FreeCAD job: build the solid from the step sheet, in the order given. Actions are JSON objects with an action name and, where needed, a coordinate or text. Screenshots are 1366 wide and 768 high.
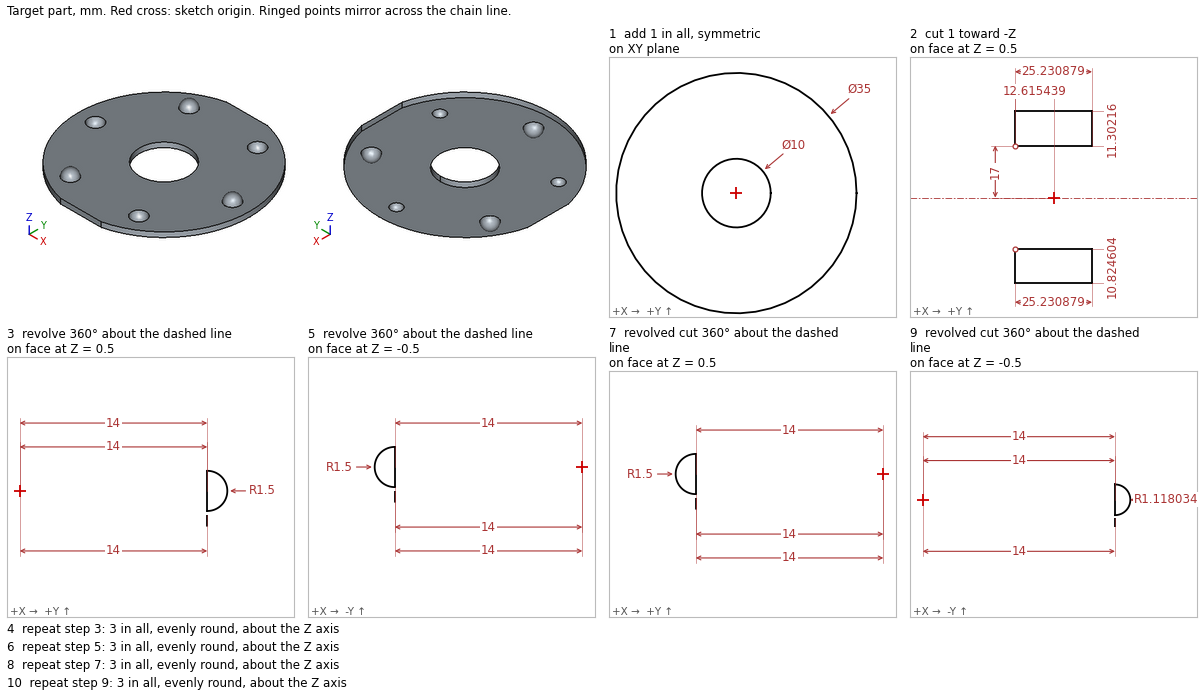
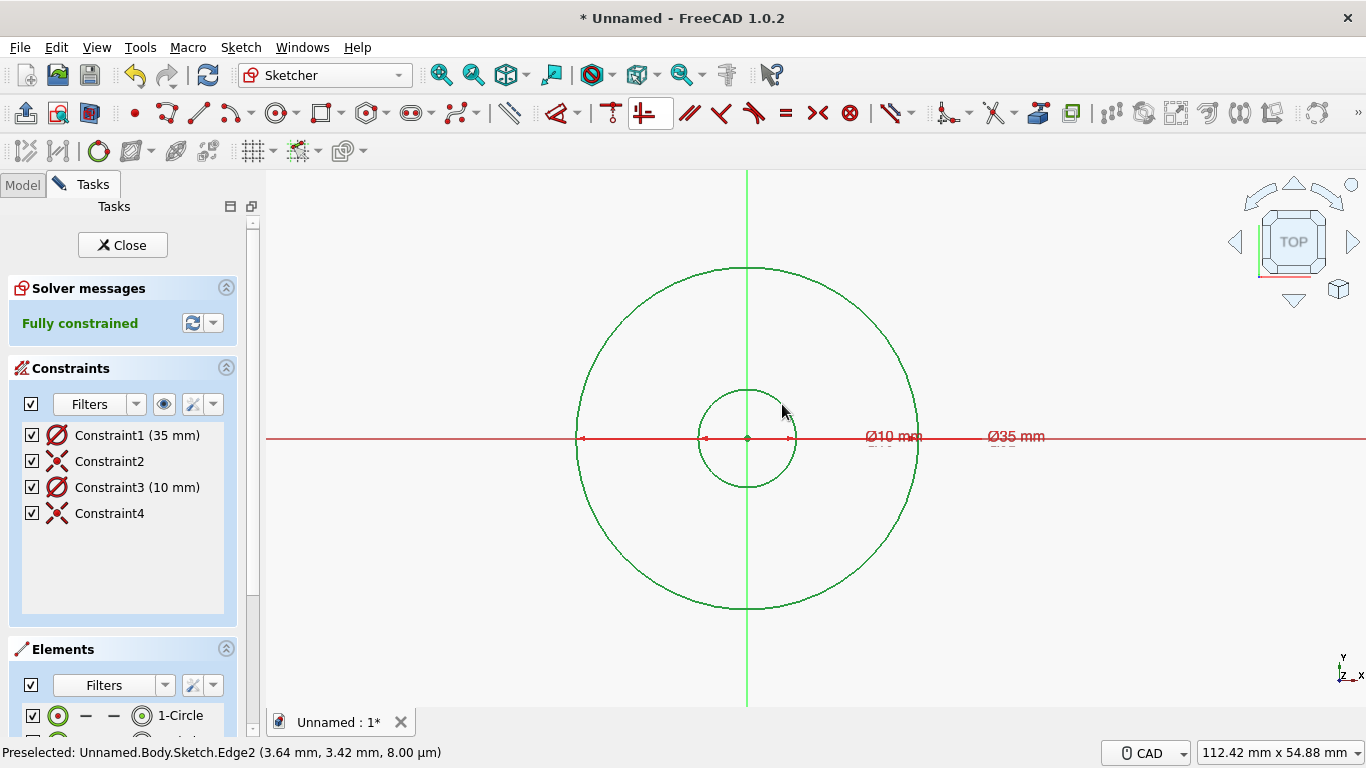
{"action": "left_click", "coordinate": [123, 245]}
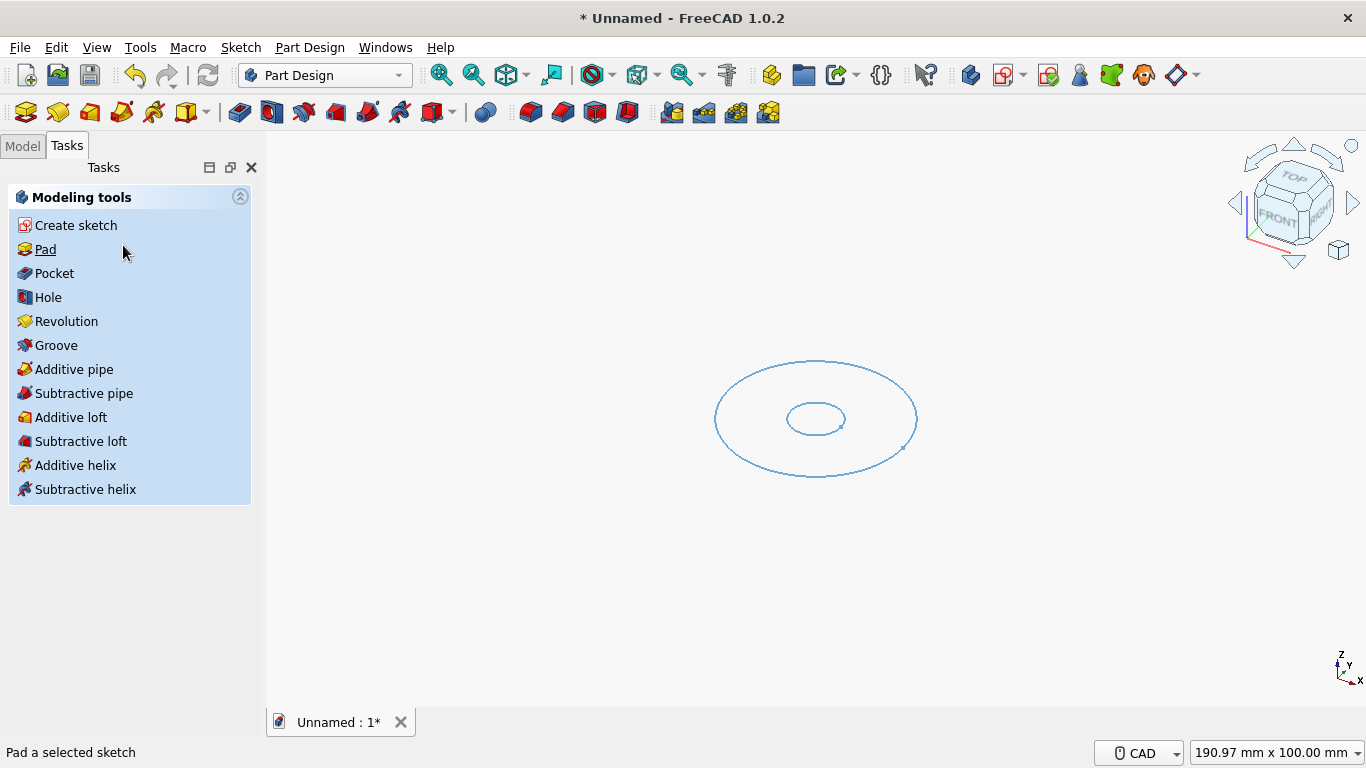
{"action": "left_click", "coordinate": [26, 112]}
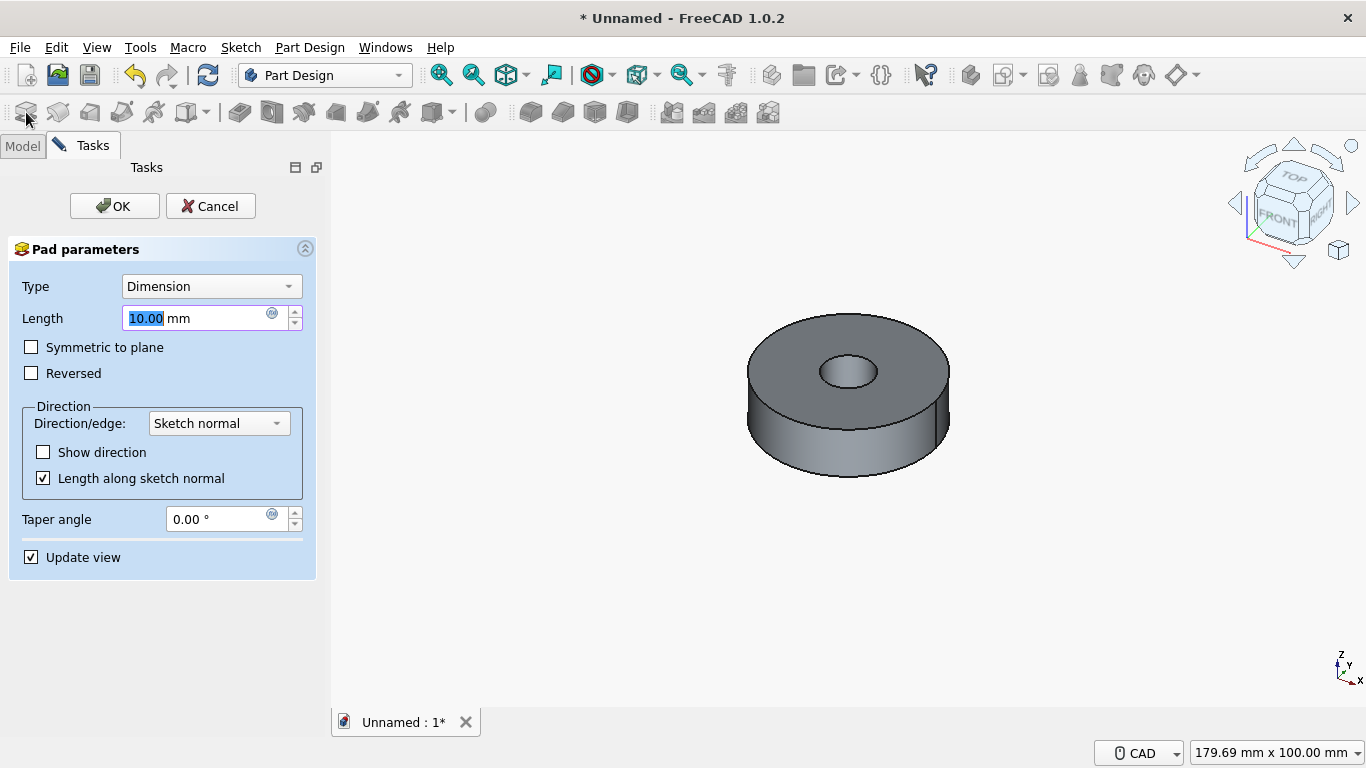
{"action": "type", "text": "1"}
{"action": "key", "text": "Tab"}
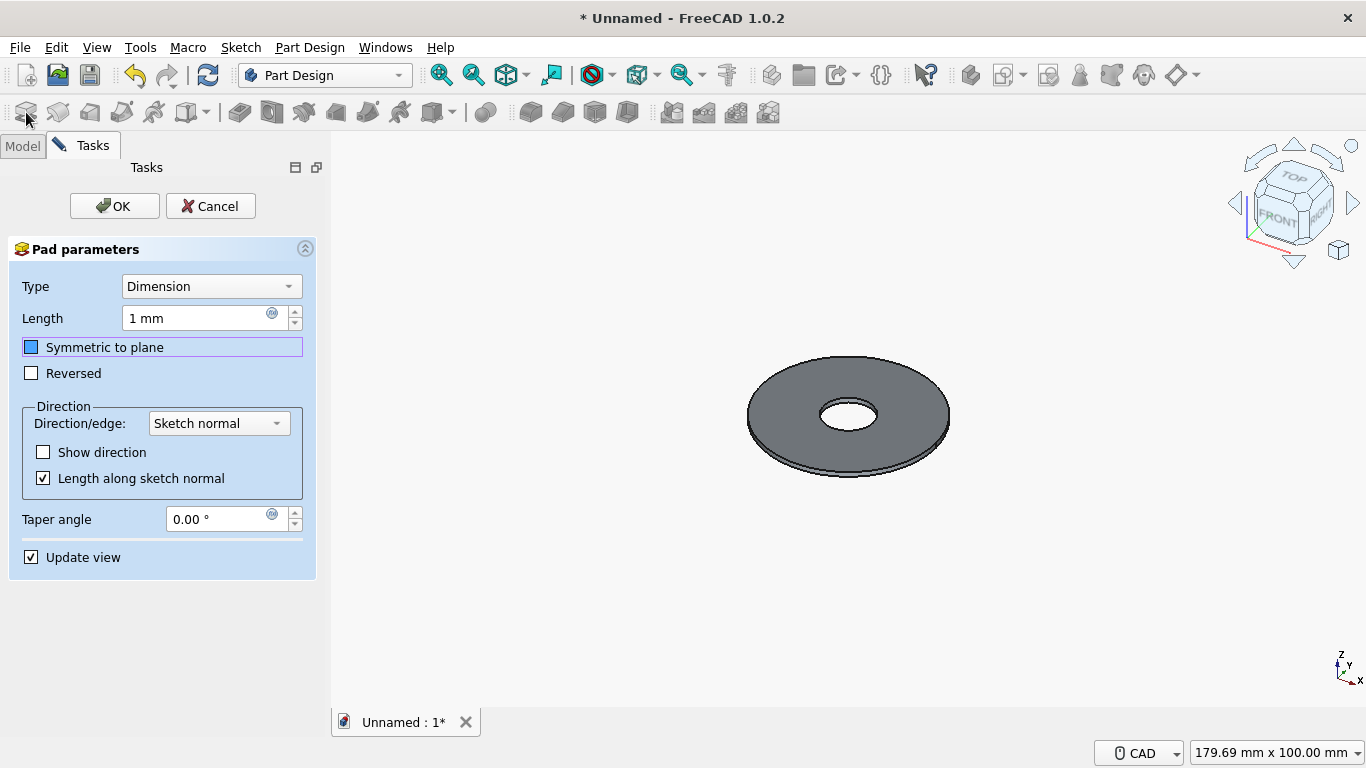
{"action": "left_click", "coordinate": [30, 347]}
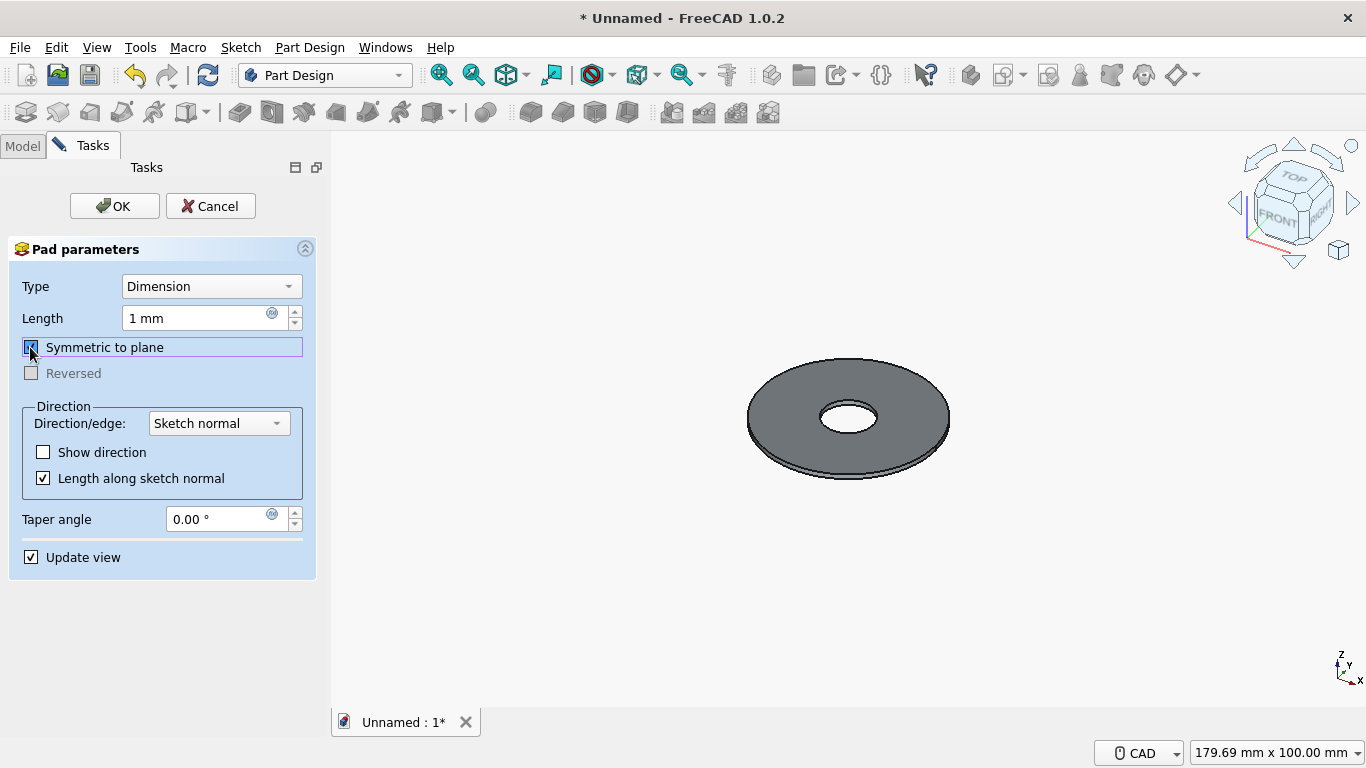
{"action": "left_click", "coordinate": [115, 206]}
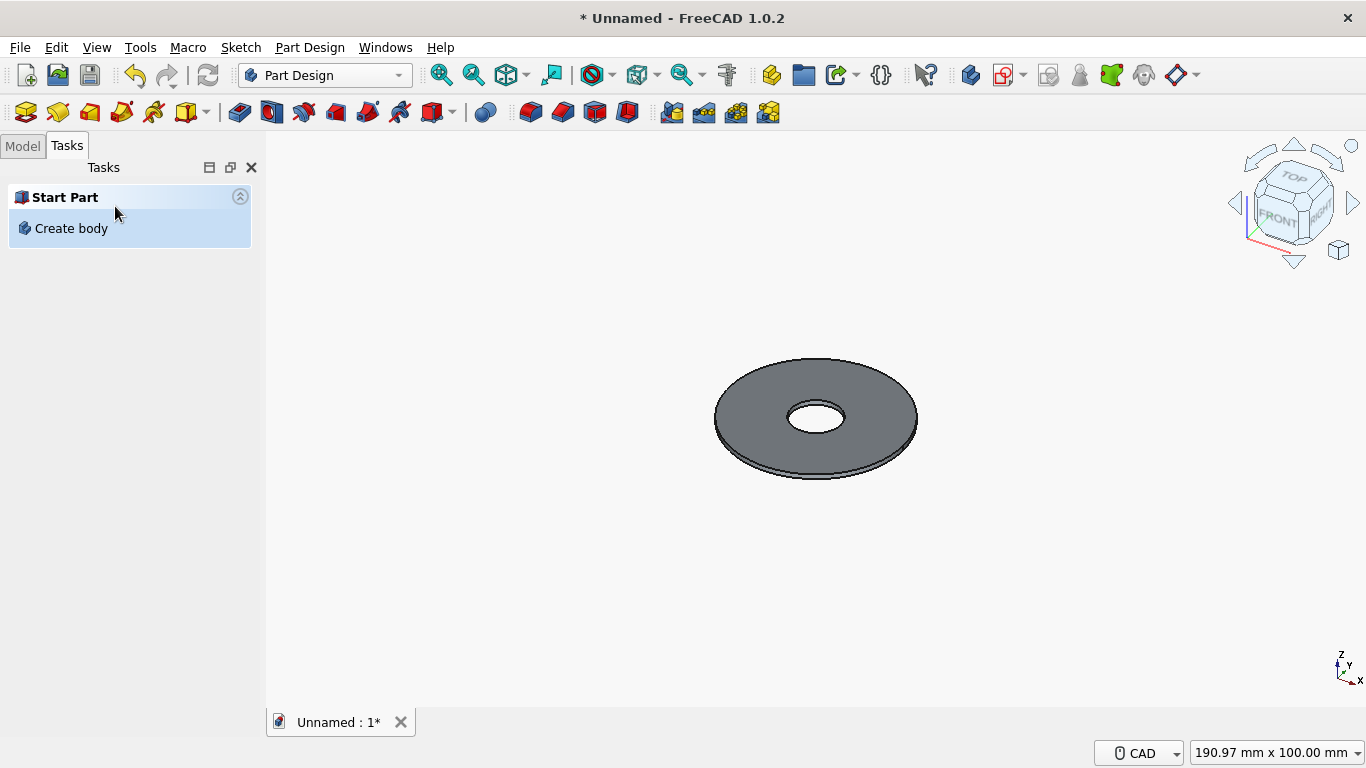
{"action": "left_click", "coordinate": [442, 76]}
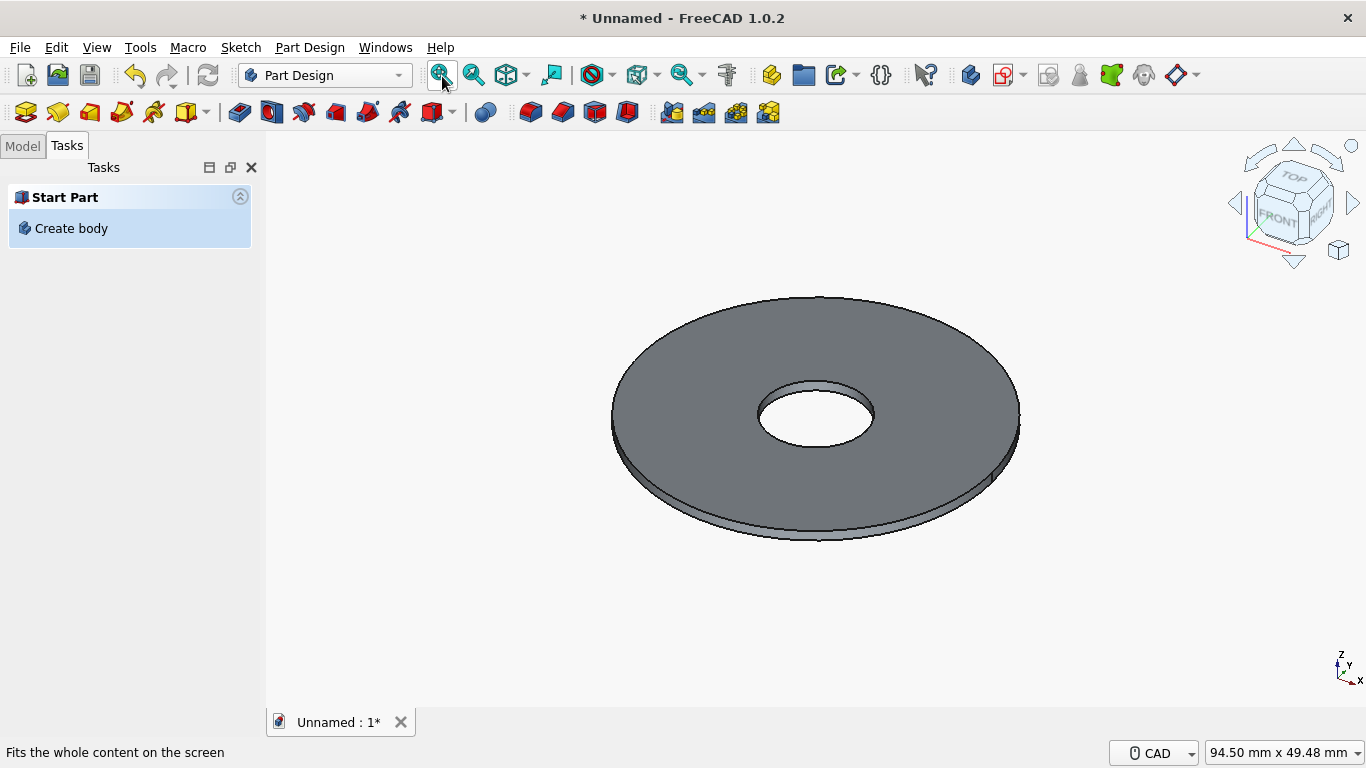
{"action": "left_click", "coordinate": [924, 372]}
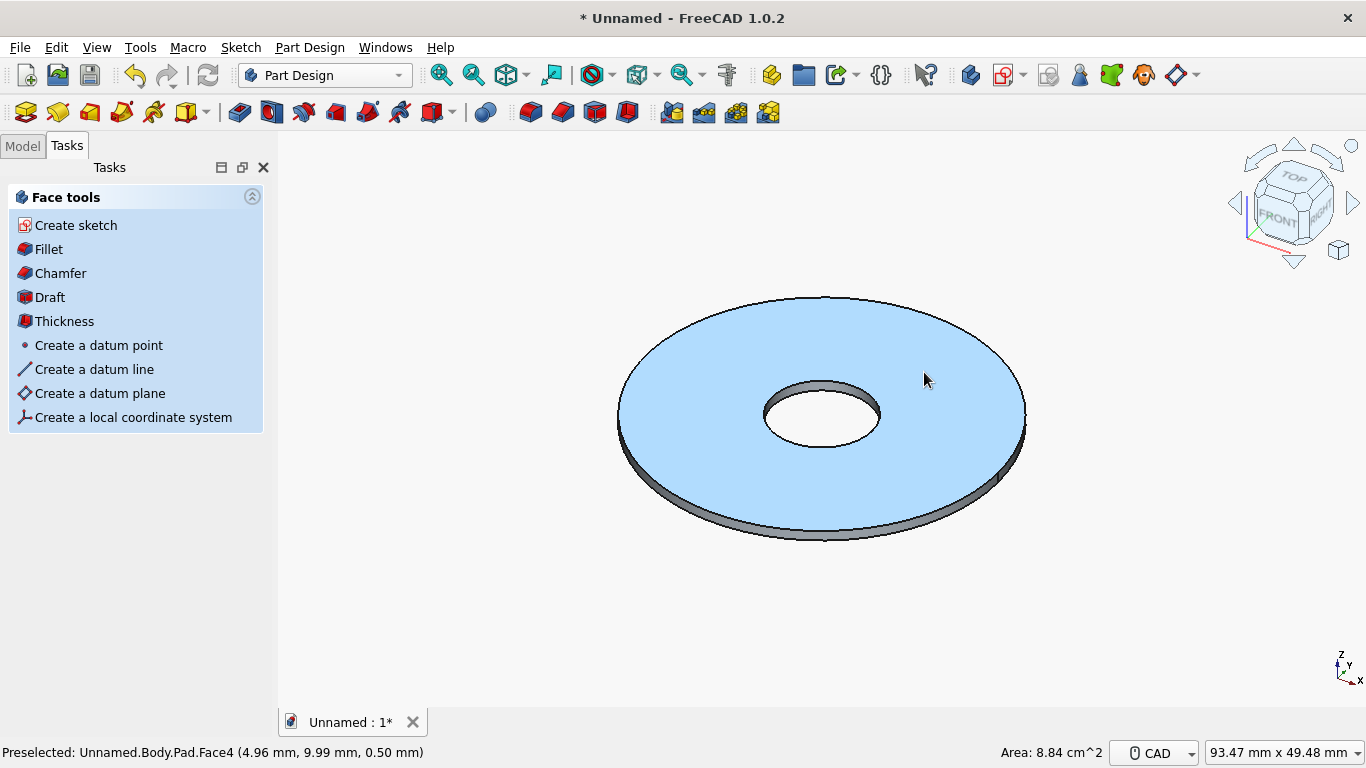
{"action": "left_click", "coordinate": [1004, 76]}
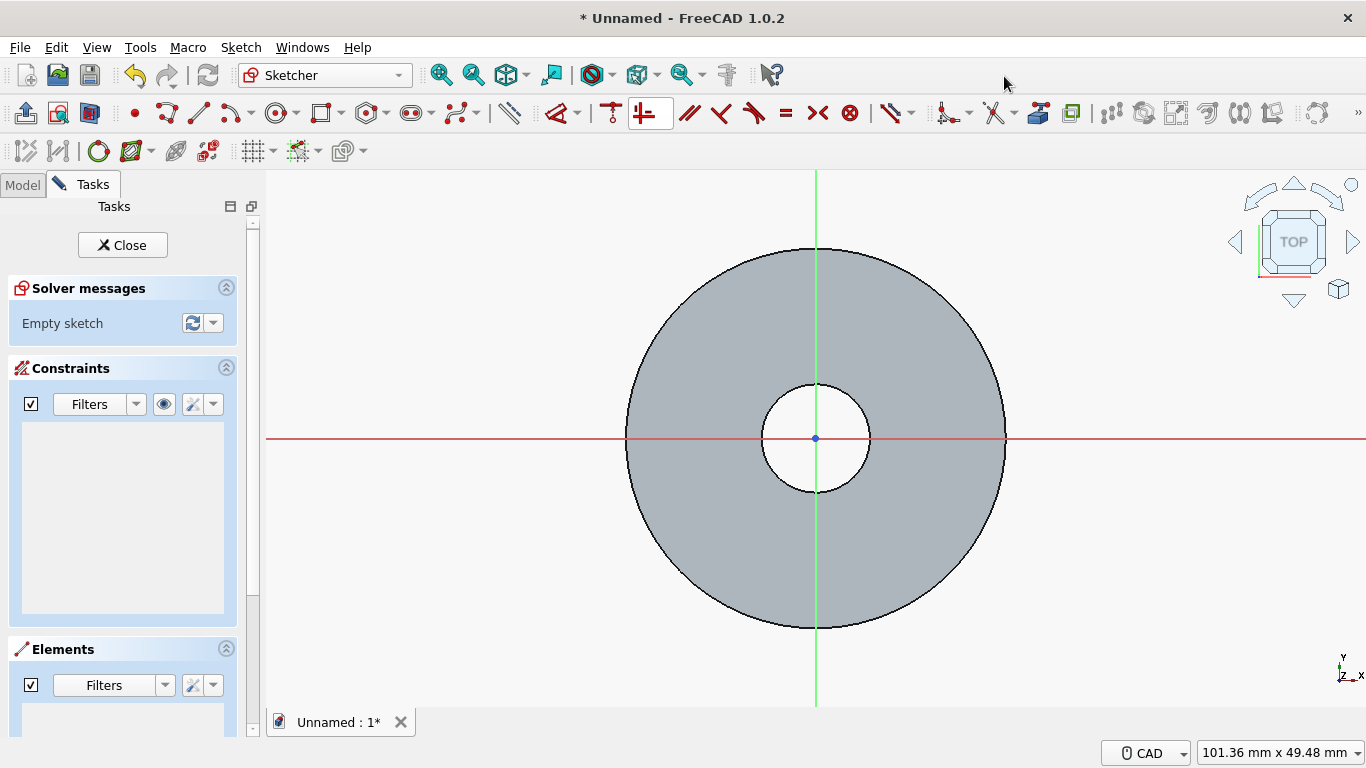
{"action": "scroll", "coordinate": [664, 442], "scroll_direction": "down", "scroll_amount": 3}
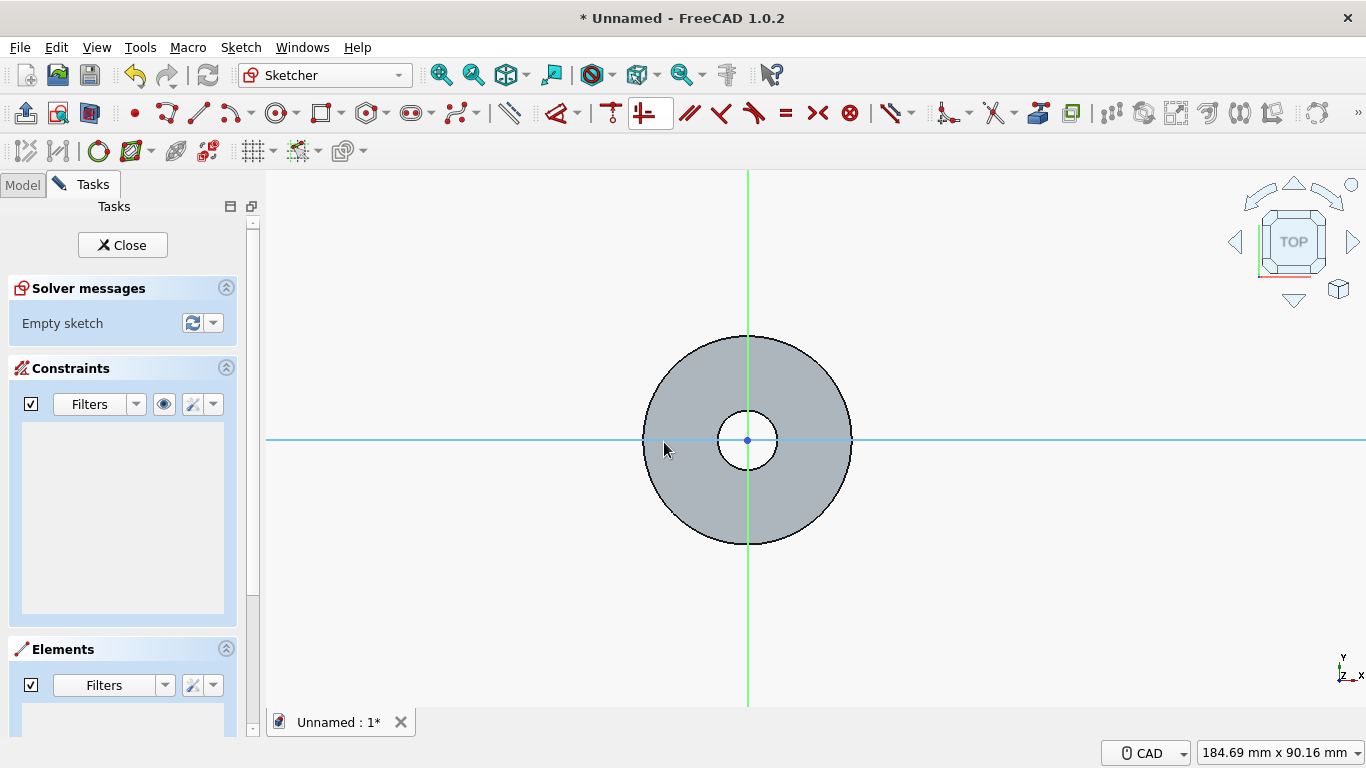
{"action": "key", "text": "g r"}